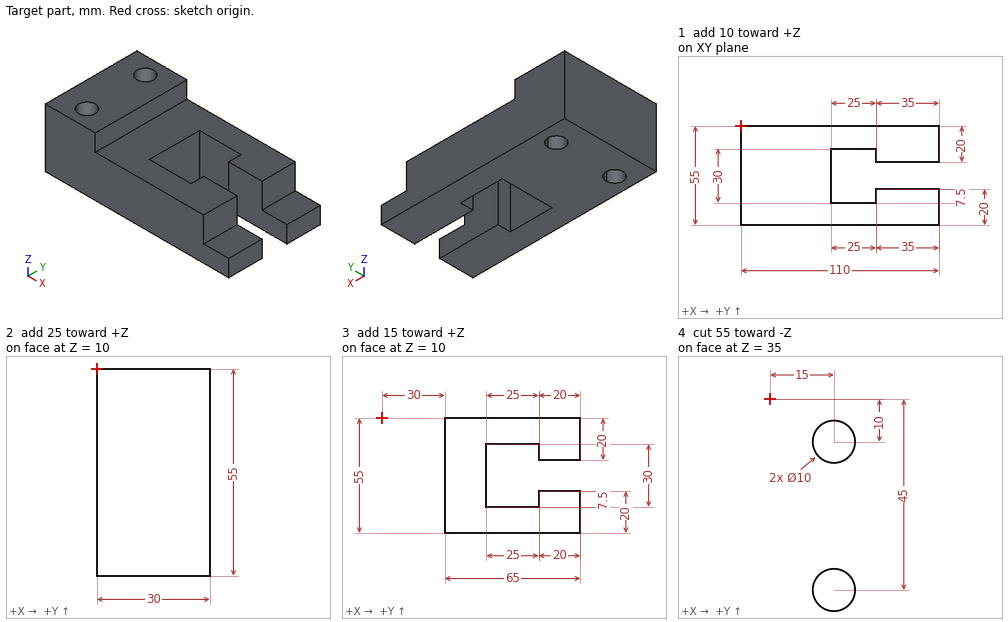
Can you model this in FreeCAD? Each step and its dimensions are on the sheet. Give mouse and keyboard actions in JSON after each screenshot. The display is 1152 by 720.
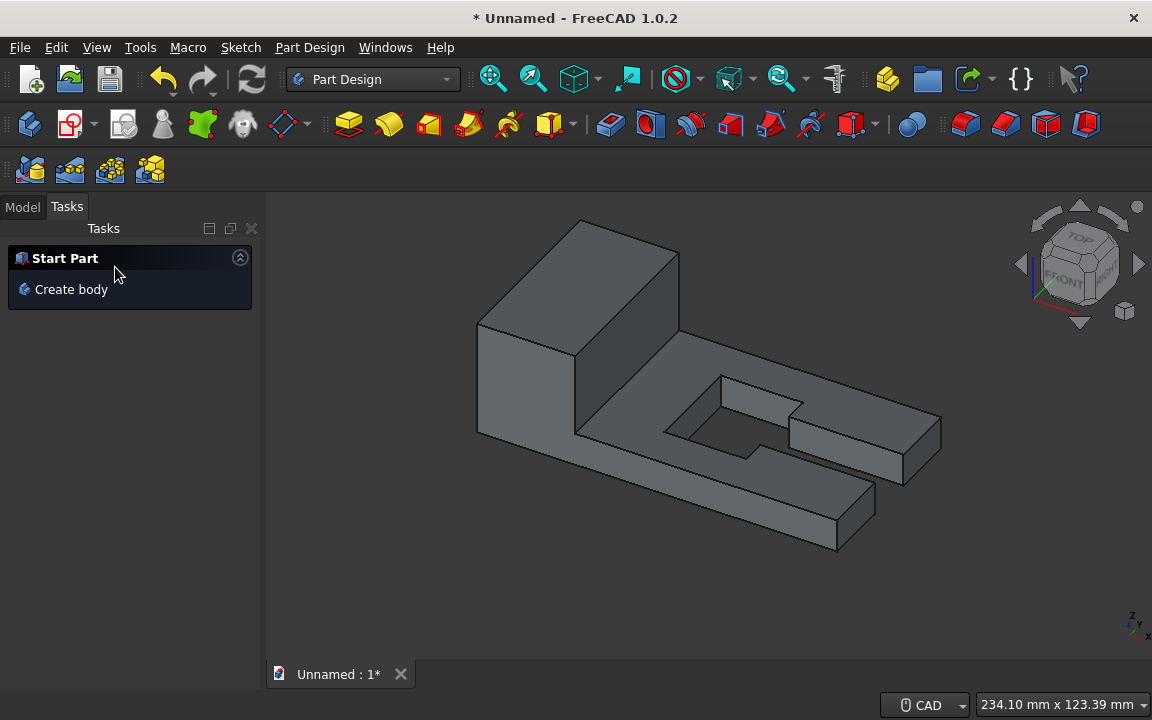
{"action": "left_click", "coordinate": [863, 420]}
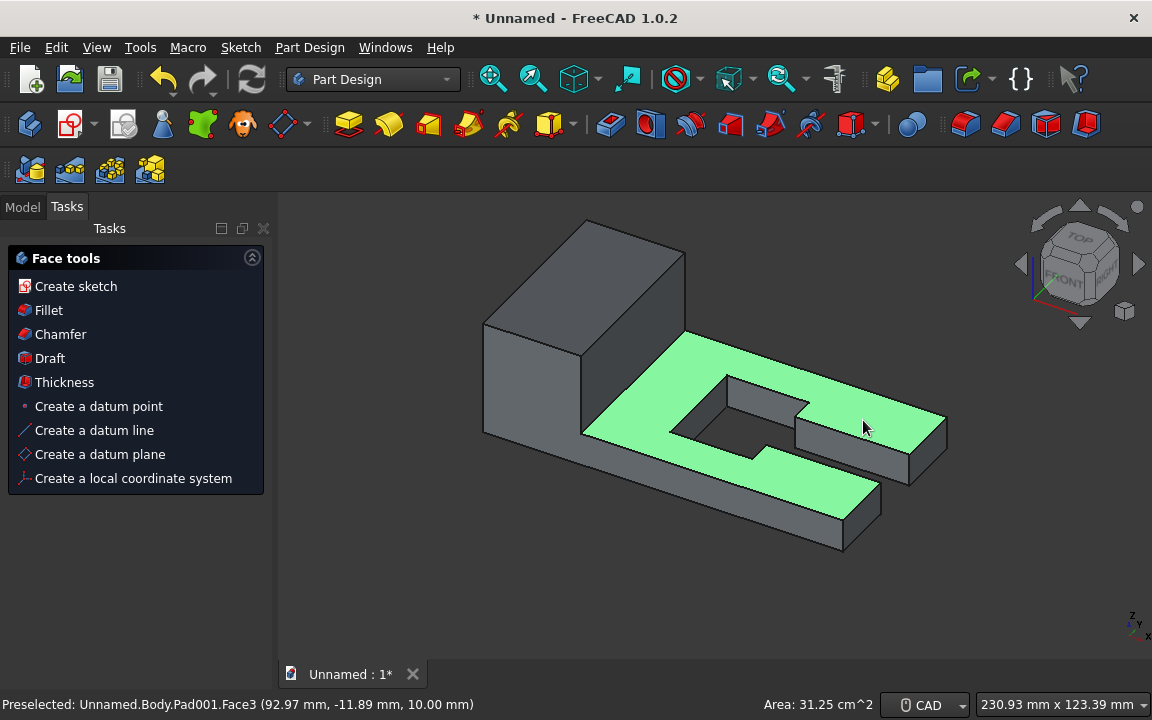
{"action": "left_click", "coordinate": [70, 124]}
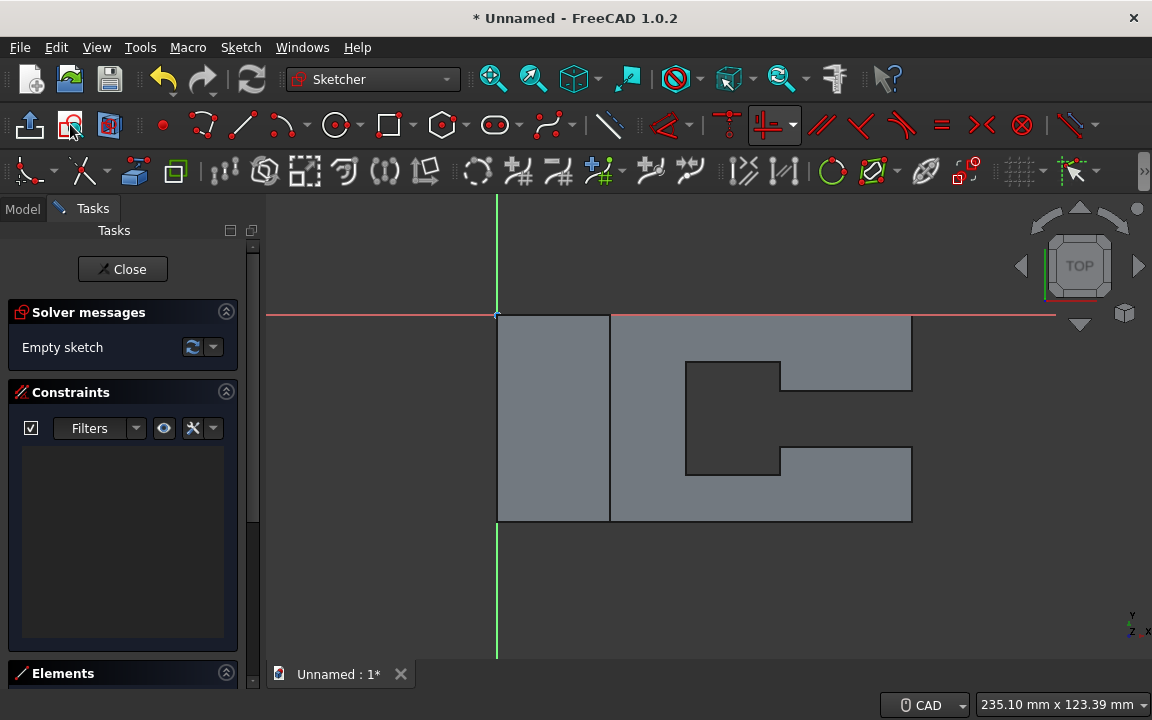
{"action": "scroll", "coordinate": [749, 403], "scroll_direction": "up", "scroll_amount": 2}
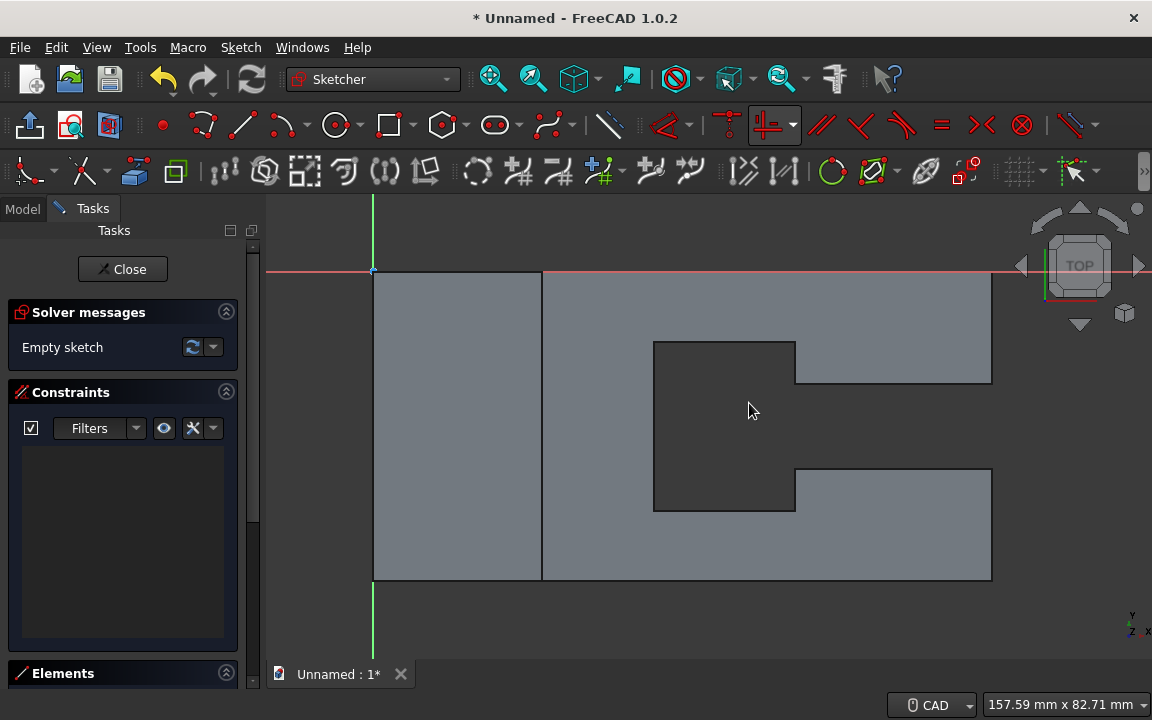
{"action": "left_click", "coordinate": [204, 126]}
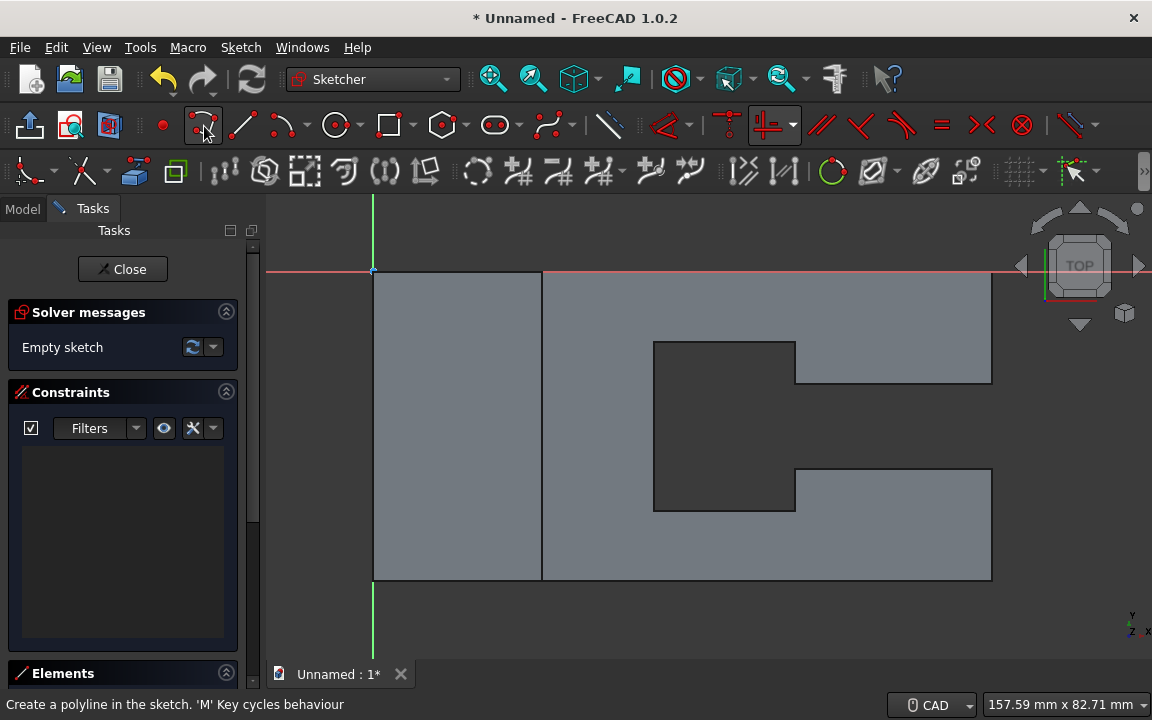
{"action": "left_click", "coordinate": [542, 272]}
{"action": "left_click", "coordinate": [542, 581]}
{"action": "left_click", "coordinate": [907, 581]}
{"action": "left_click", "coordinate": [907, 469]}
{"action": "left_click", "coordinate": [795, 469]}
{"action": "left_click", "coordinate": [795, 511]}
{"action": "left_click", "coordinate": [654, 511]}
{"action": "left_click", "coordinate": [654, 342]}
{"action": "left_click", "coordinate": [795, 342]}
{"action": "left_click", "coordinate": [795, 384]}
{"action": "left_click", "coordinate": [907, 384]}
{"action": "left_click", "coordinate": [907, 281]}
{"action": "left_click", "coordinate": [542, 272]}
{"action": "key", "text": "Escape"}
{"action": "key", "text": "Escape"}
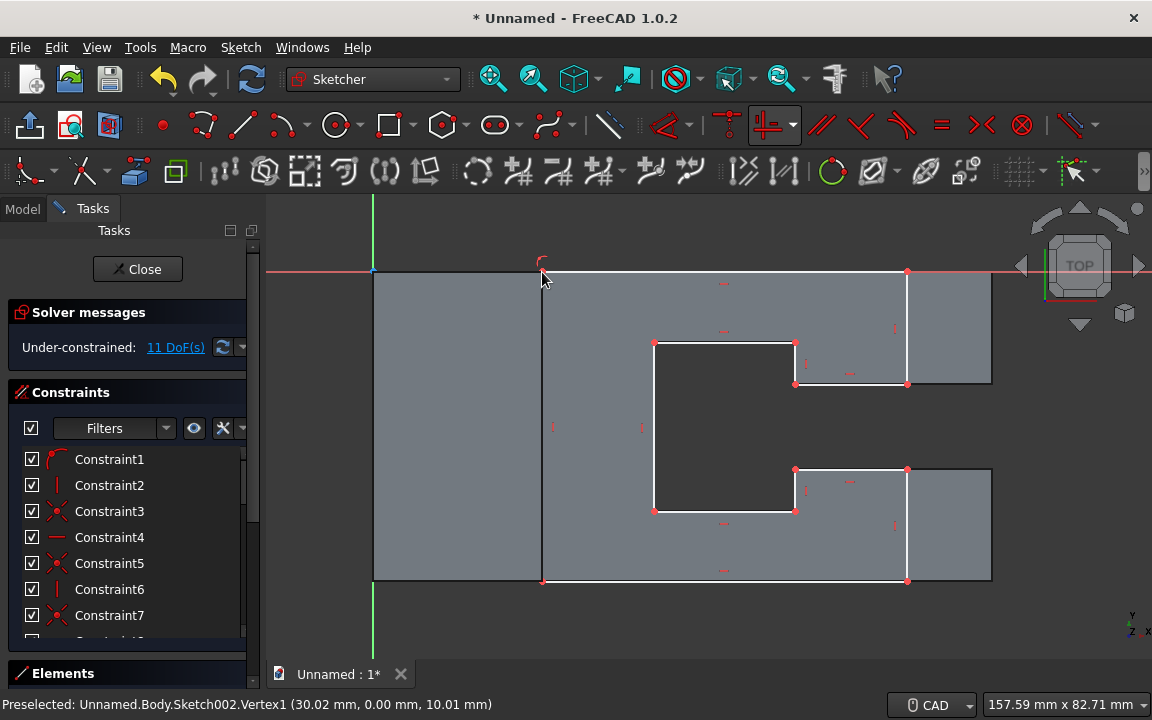
{"action": "left_click", "coordinate": [664, 126]}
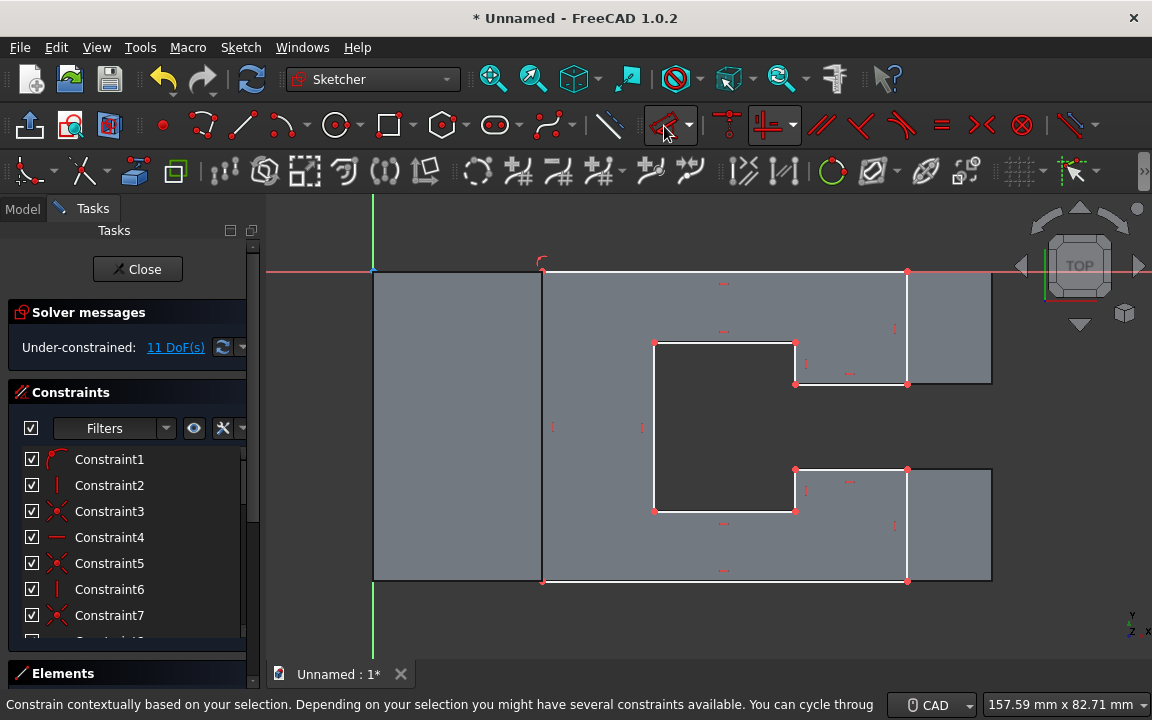
{"action": "left_click", "coordinate": [542, 365]}
{"action": "left_click", "coordinate": [508, 427]}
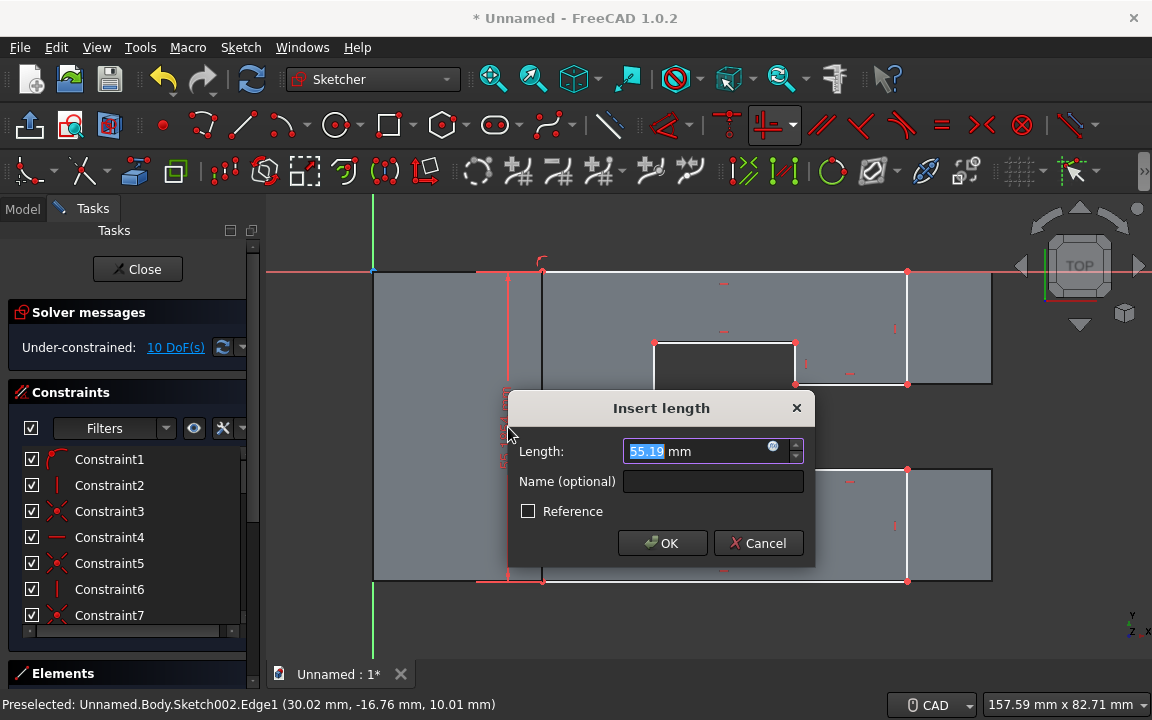
{"action": "type", "text": "55"}
{"action": "key", "text": "Return"}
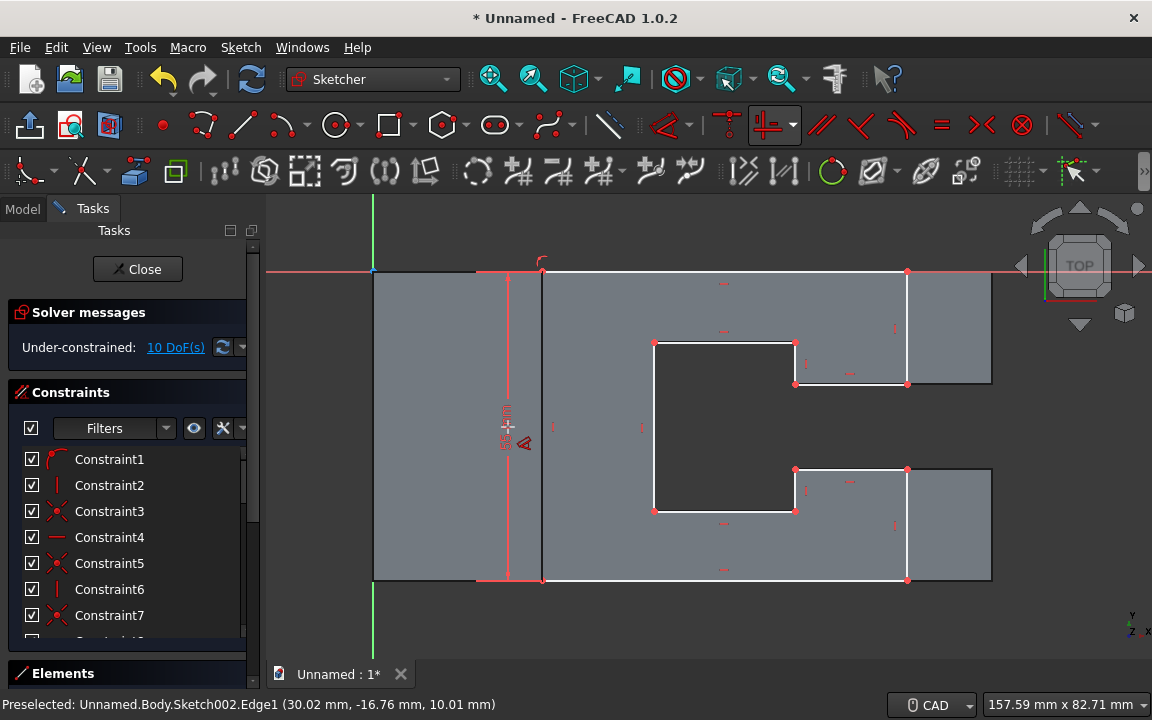
{"action": "left_click", "coordinate": [651, 581]}
{"action": "left_click", "coordinate": [724, 615]}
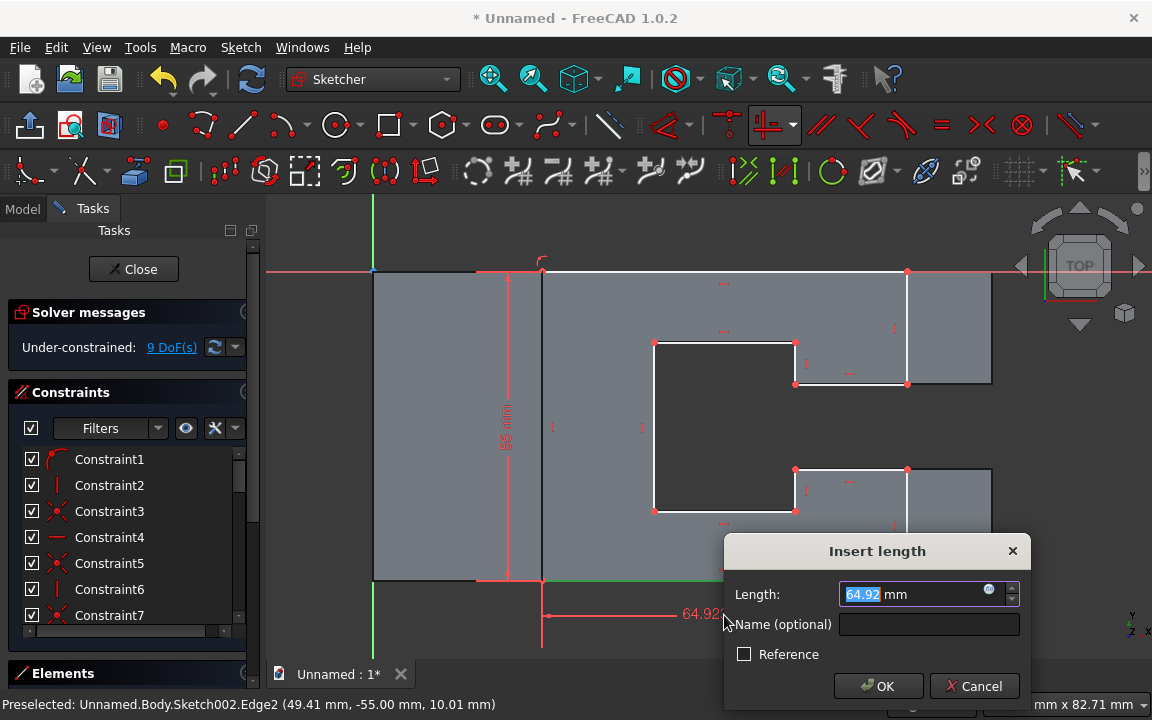
{"action": "type", "text": "65"}
{"action": "key", "text": "Return"}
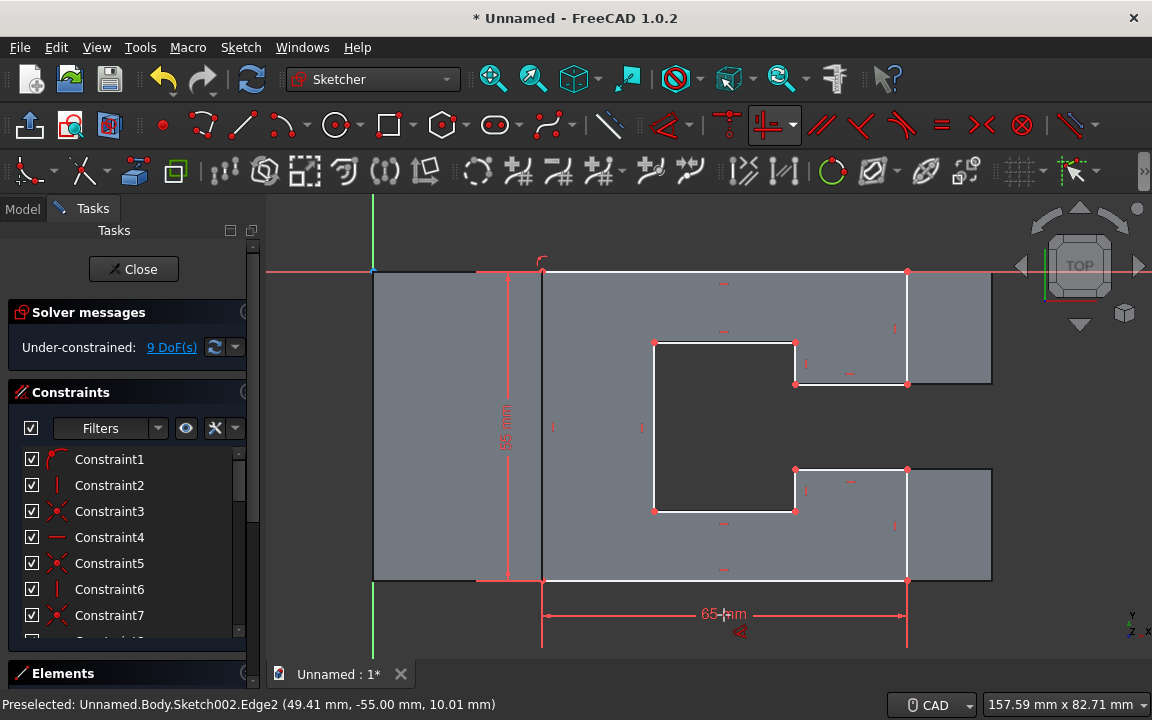
{"action": "left_click", "coordinate": [907, 548]}
{"action": "left_click", "coordinate": [941, 525]}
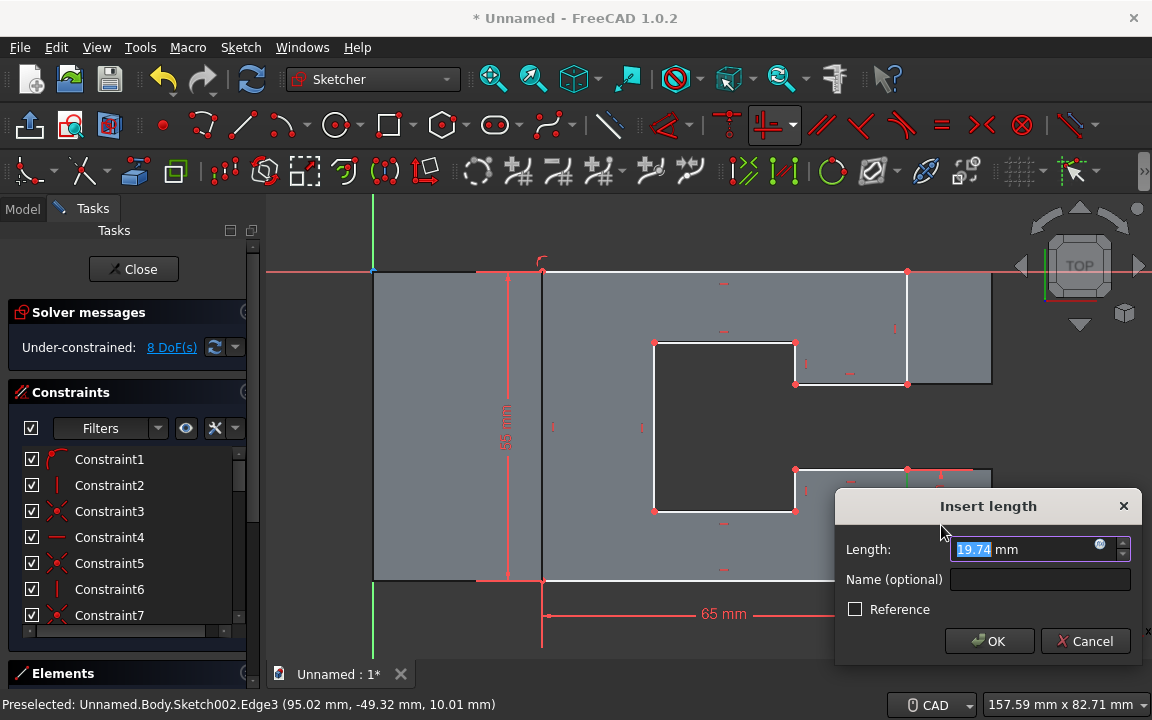
{"action": "type", "text": "20"}
{"action": "key", "text": "Return"}